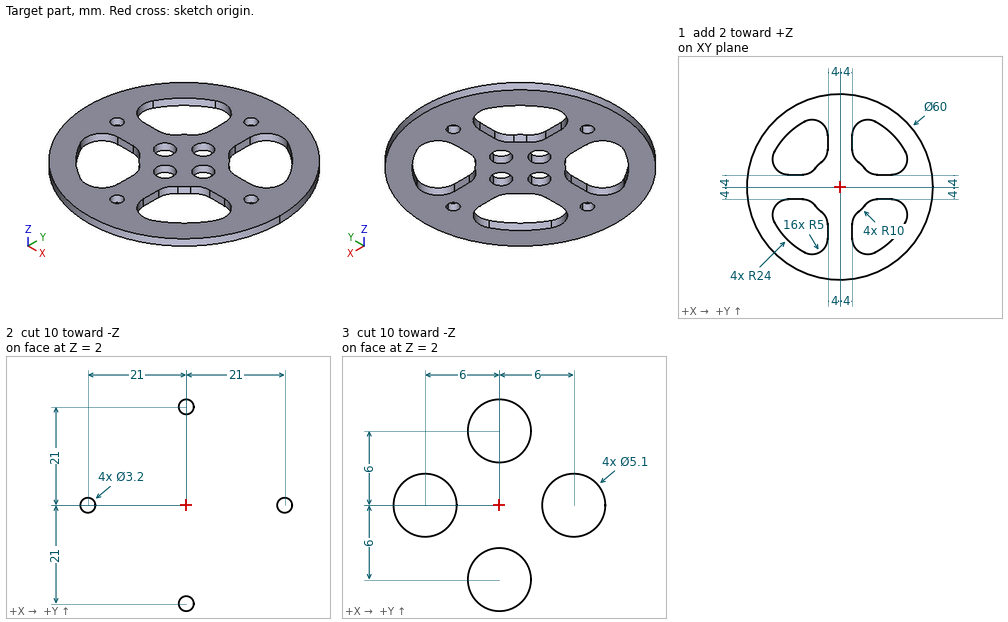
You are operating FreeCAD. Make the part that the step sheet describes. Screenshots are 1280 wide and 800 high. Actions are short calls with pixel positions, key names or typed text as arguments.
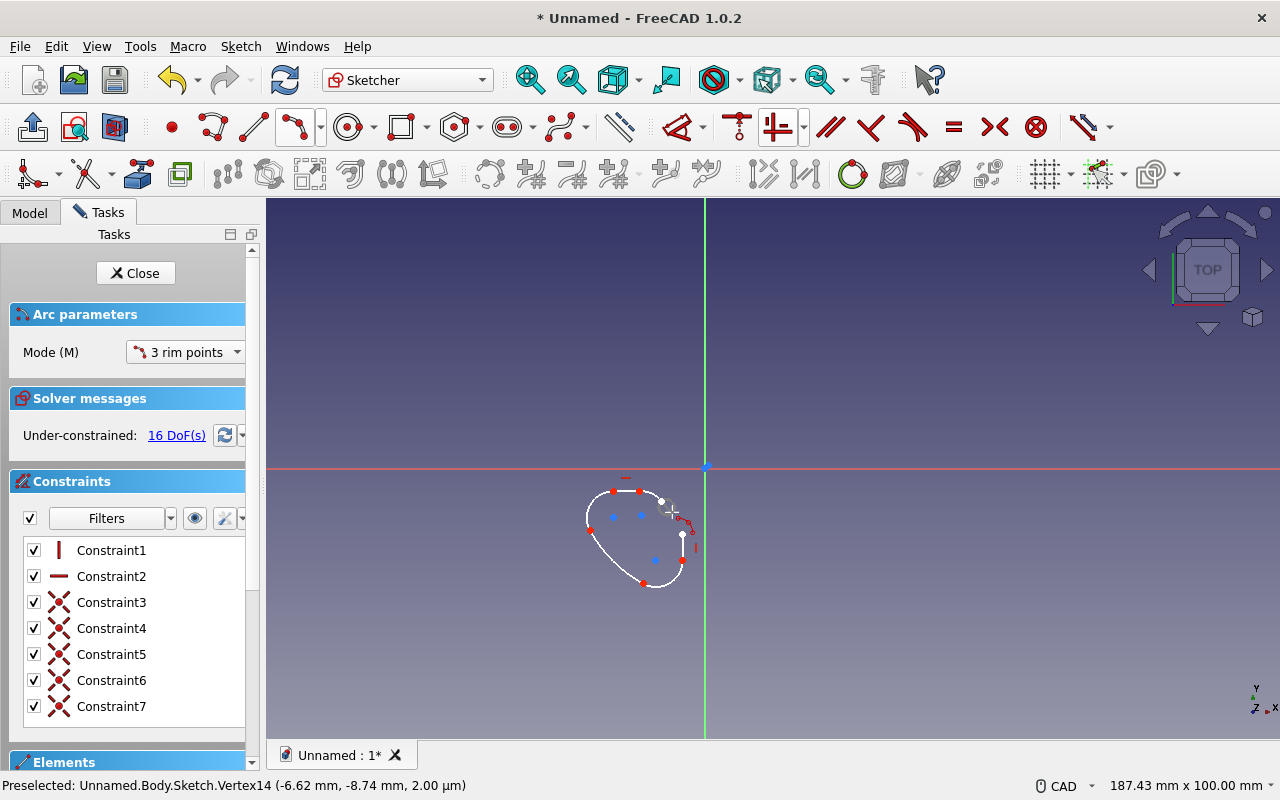
scroll(666, 507, up, 17)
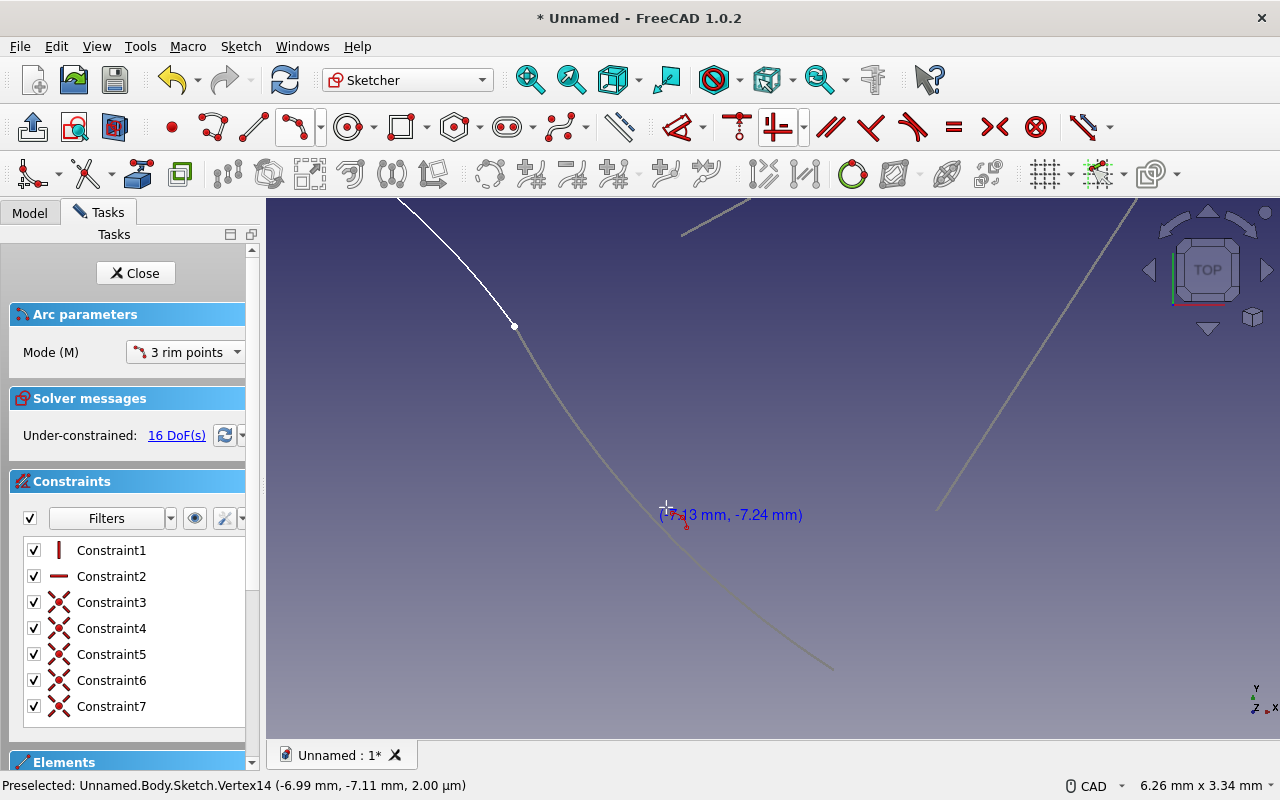
click(664, 494)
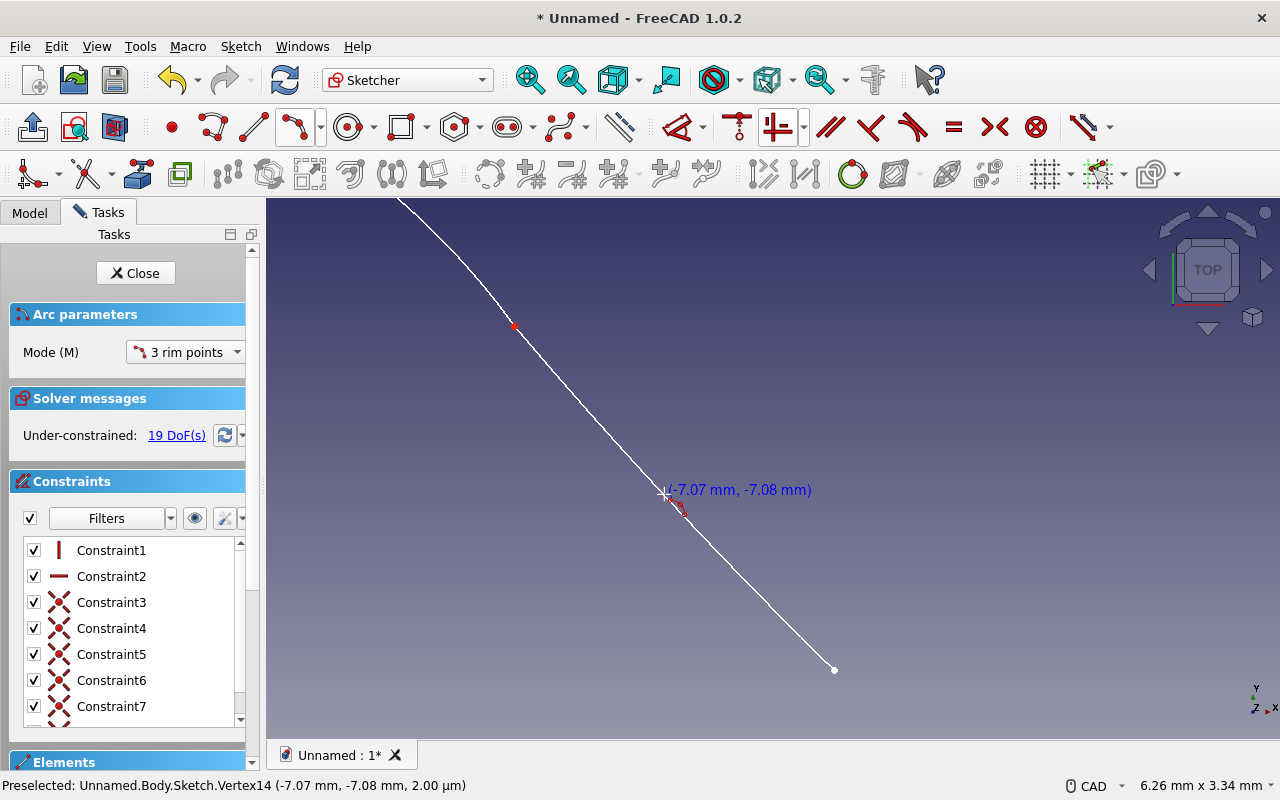
scroll(658, 516, down, 16)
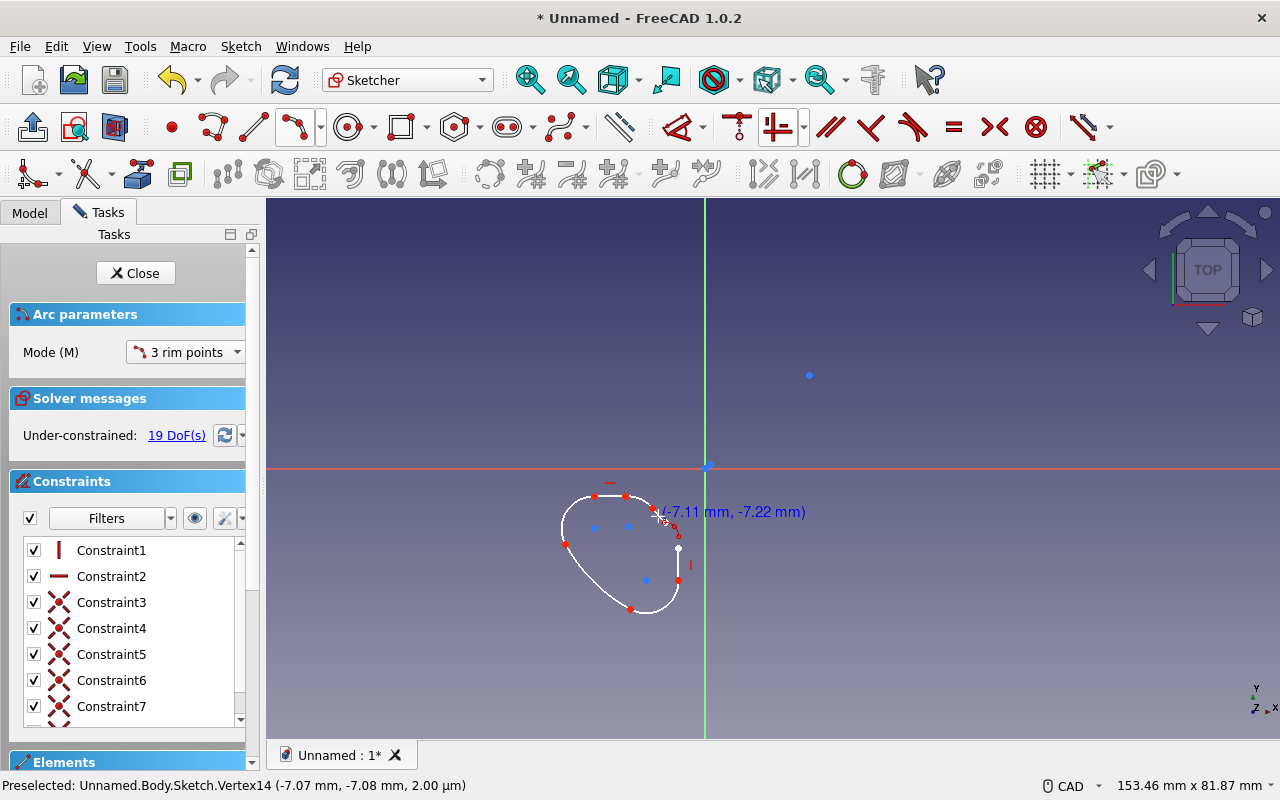
click(666, 523)
click(678, 549)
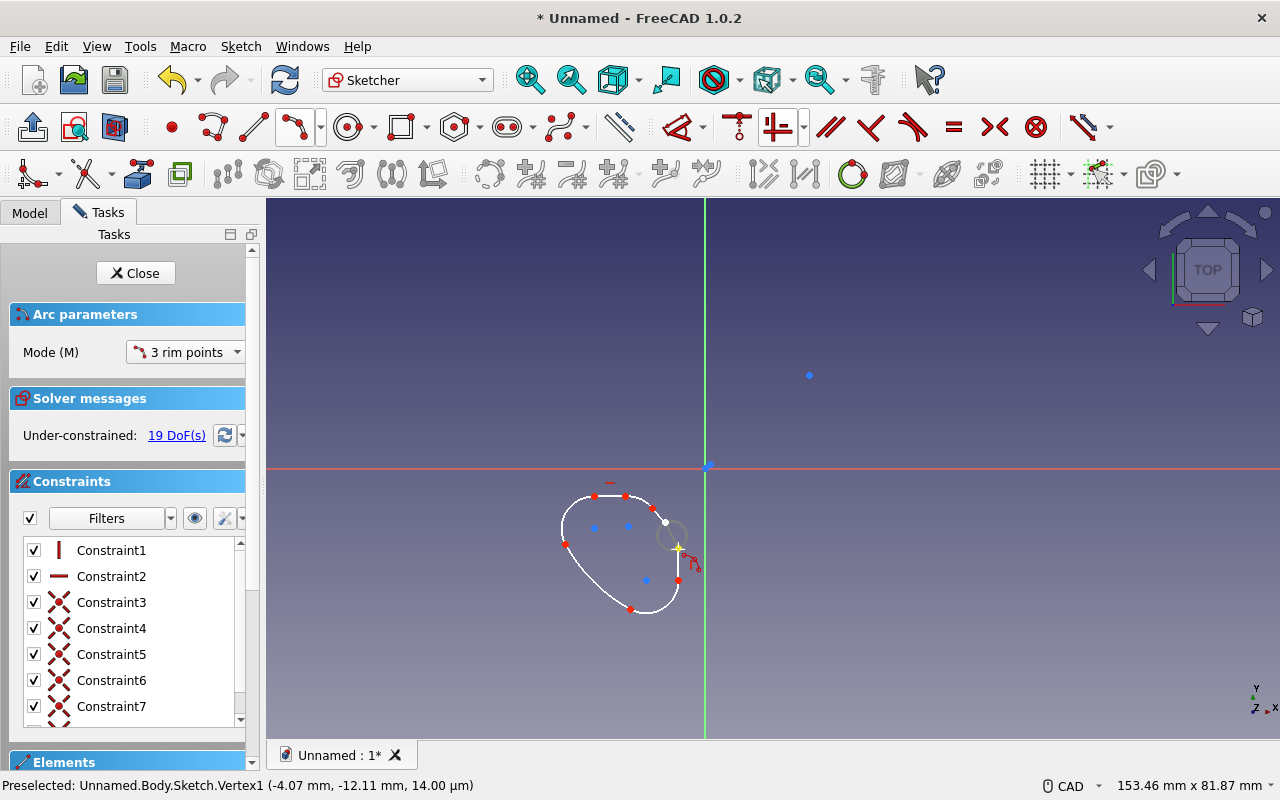
scroll(675, 533, up, 8)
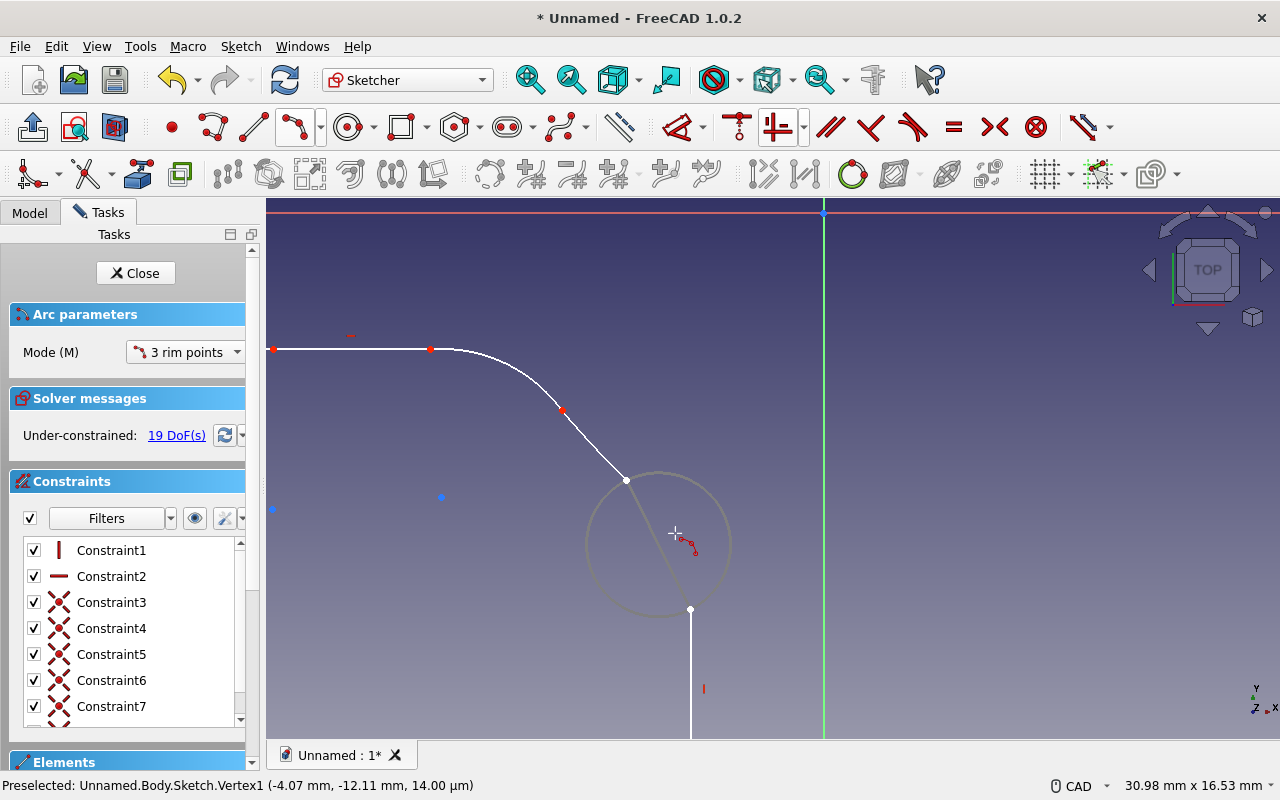
click(675, 533)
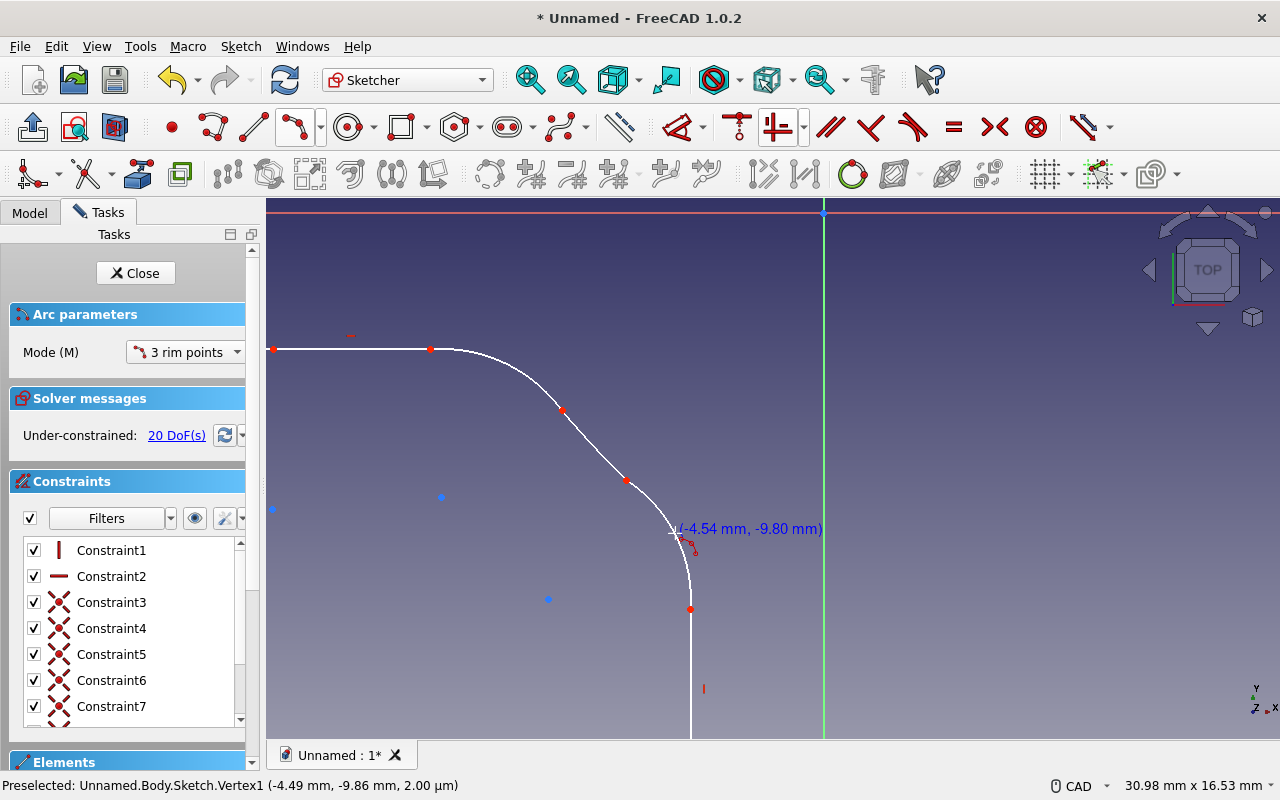
click(254, 128)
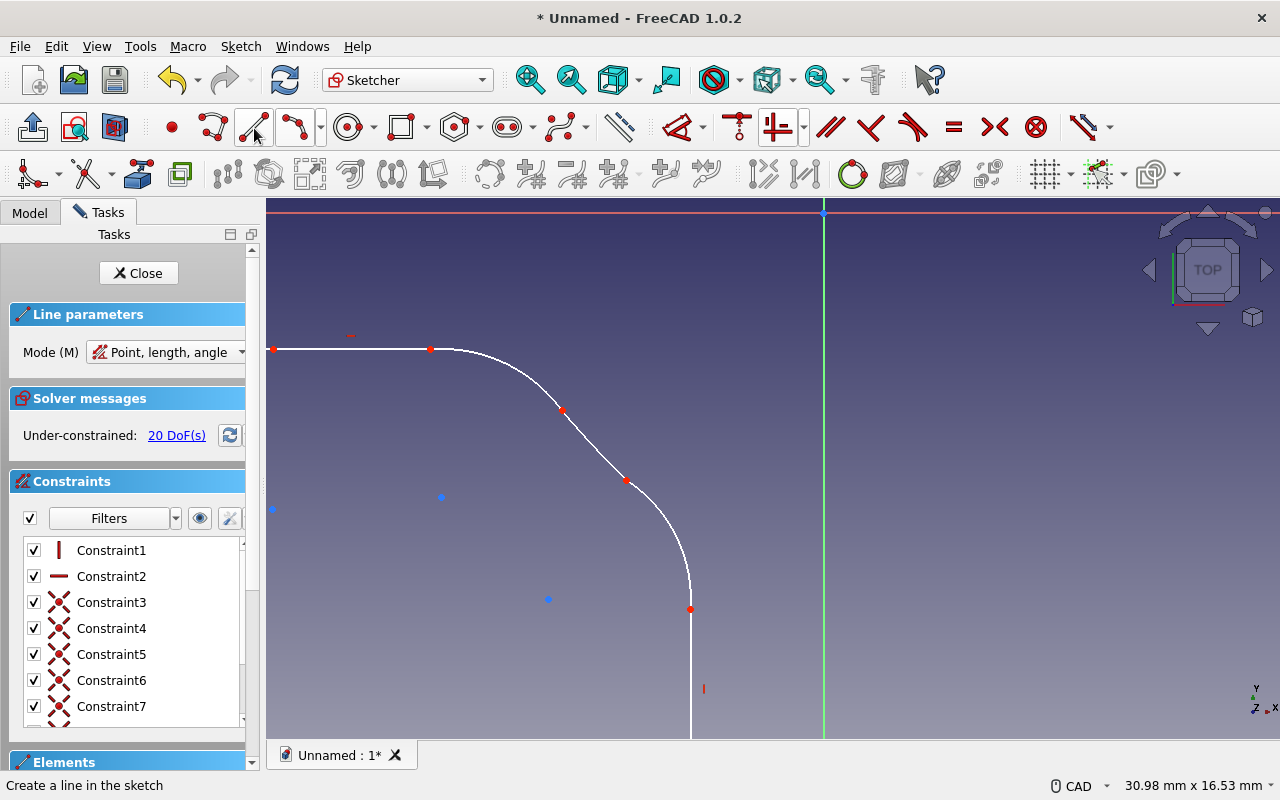
scroll(681, 519, down, 9)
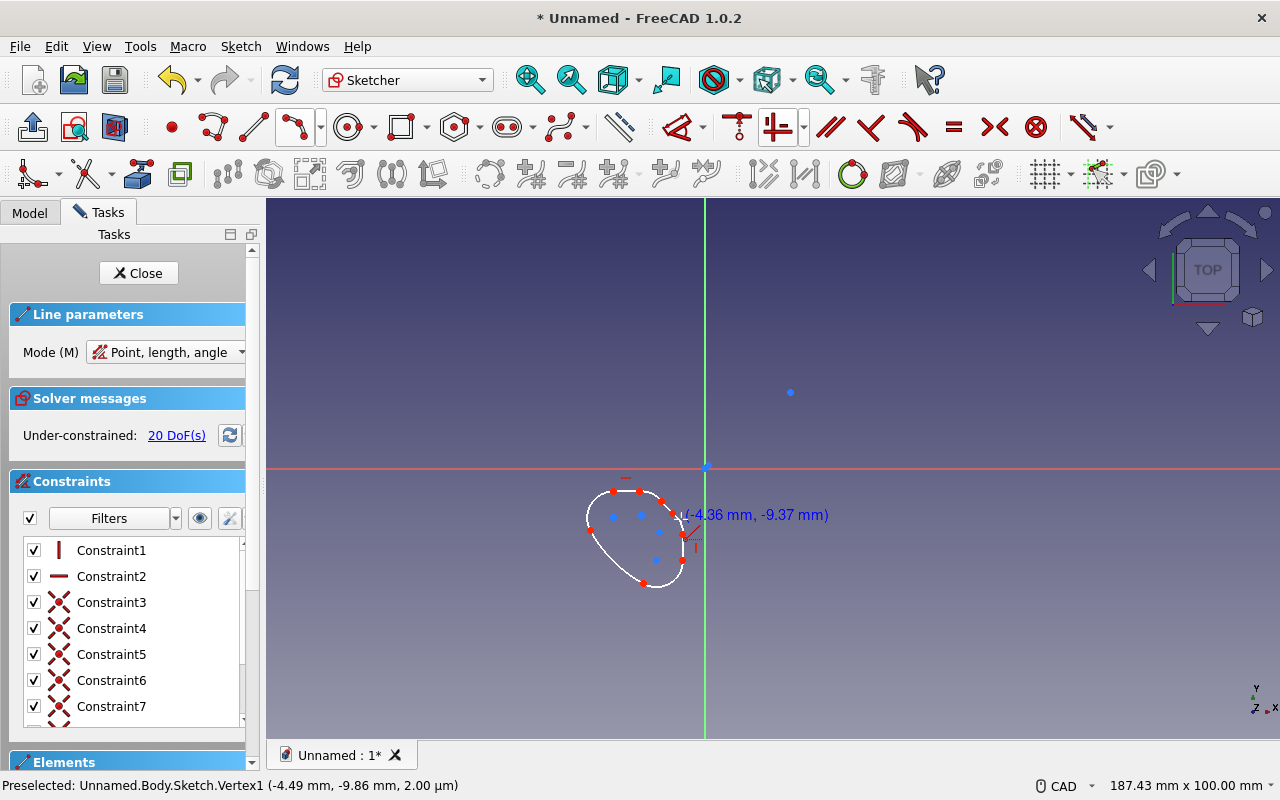
click(770, 491)
click(795, 491)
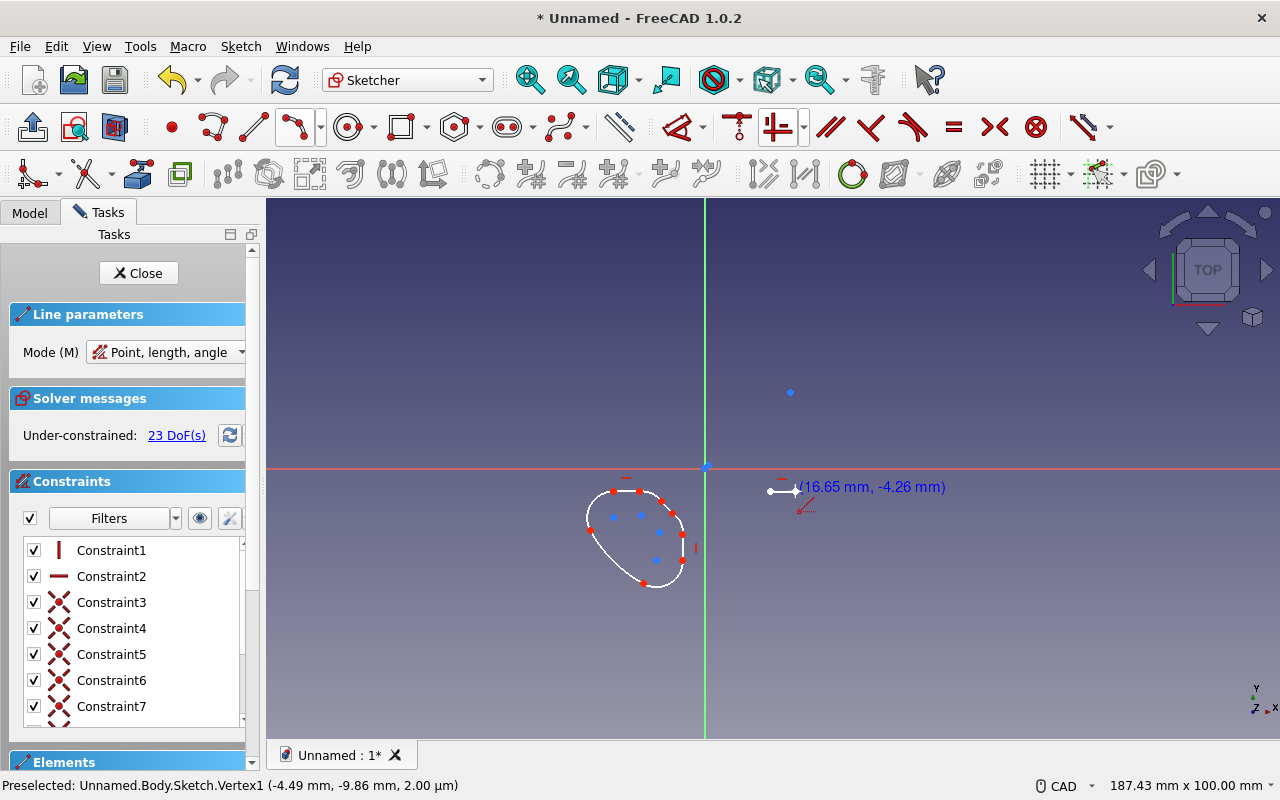
click(727, 559)
click(727, 534)